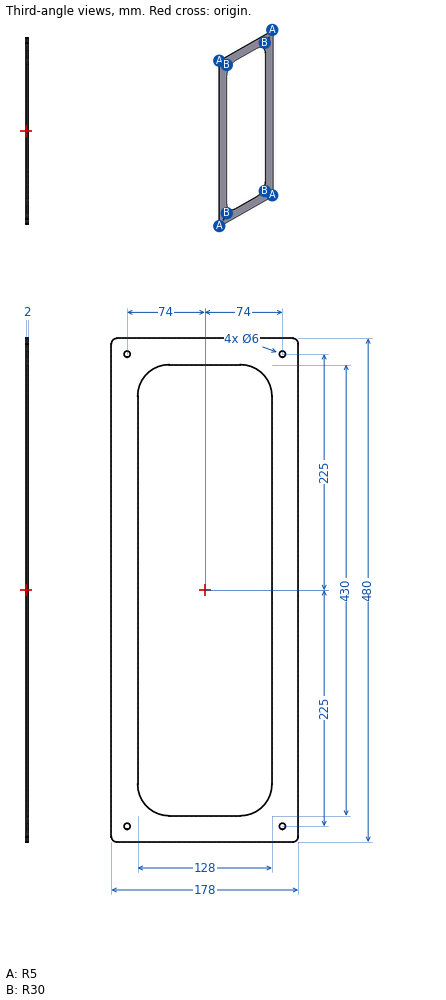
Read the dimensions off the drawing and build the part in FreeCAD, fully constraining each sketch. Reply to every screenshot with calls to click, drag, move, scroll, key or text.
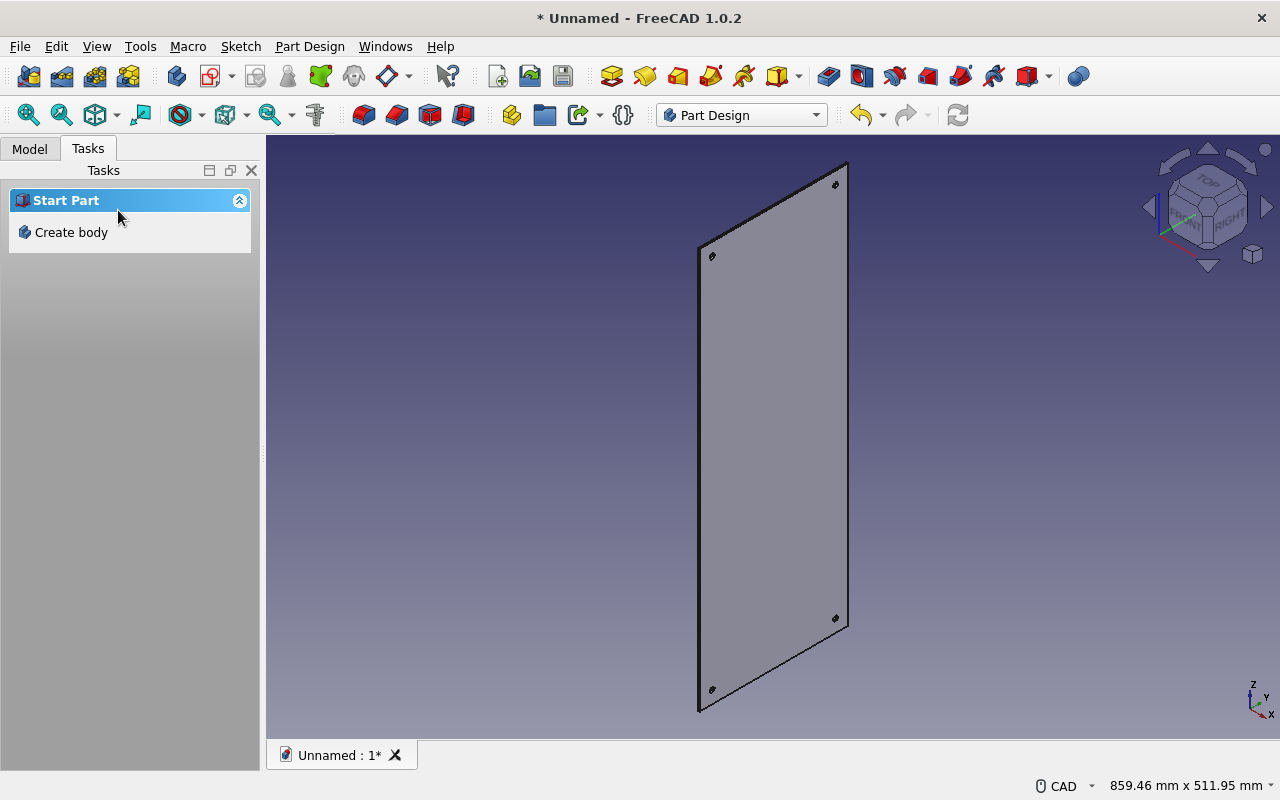
key(2)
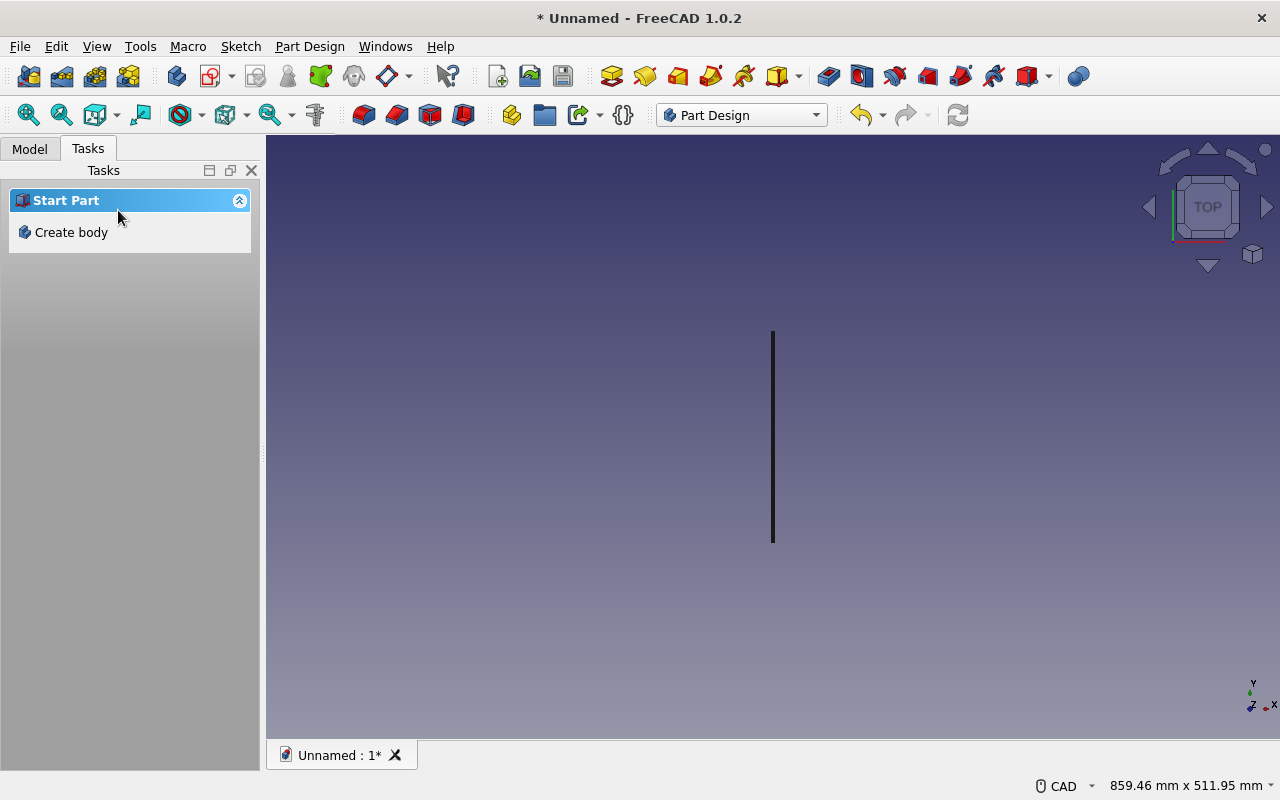
click(29, 116)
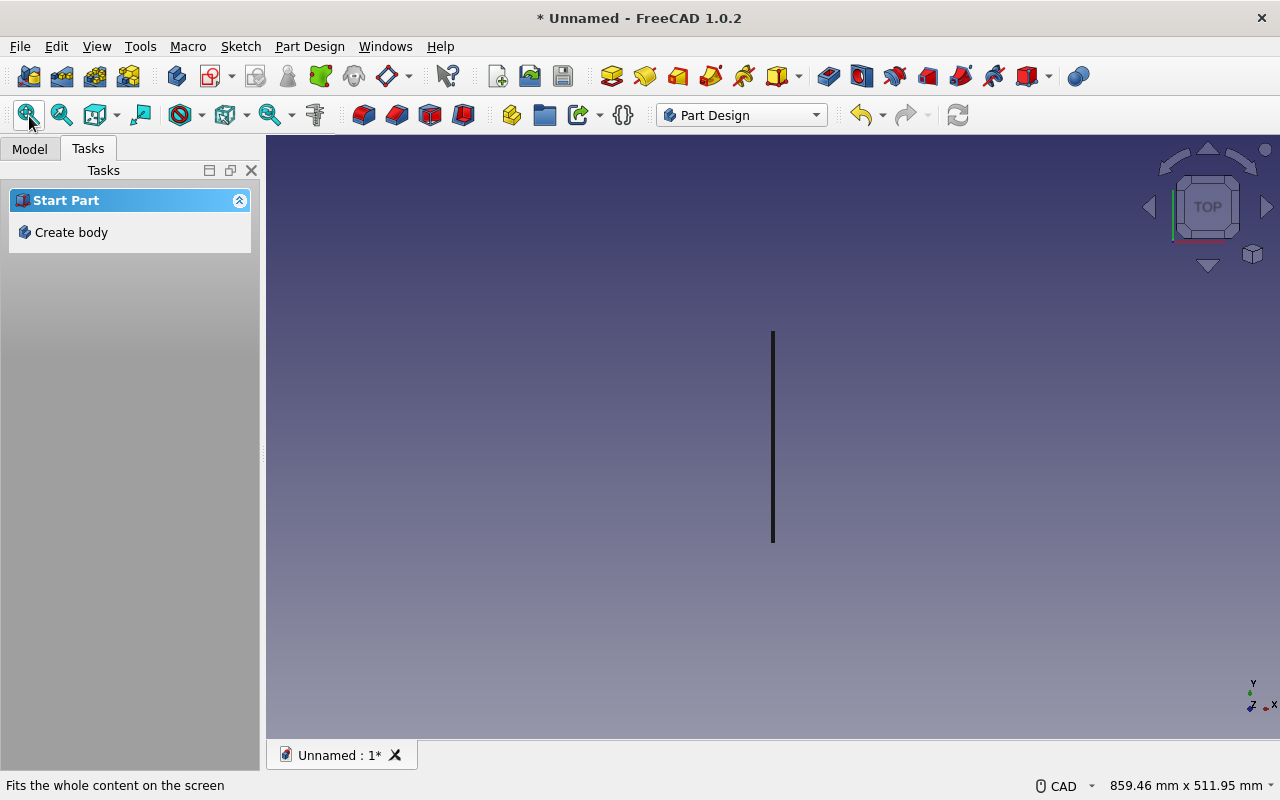
scroll(773, 331, up, 15)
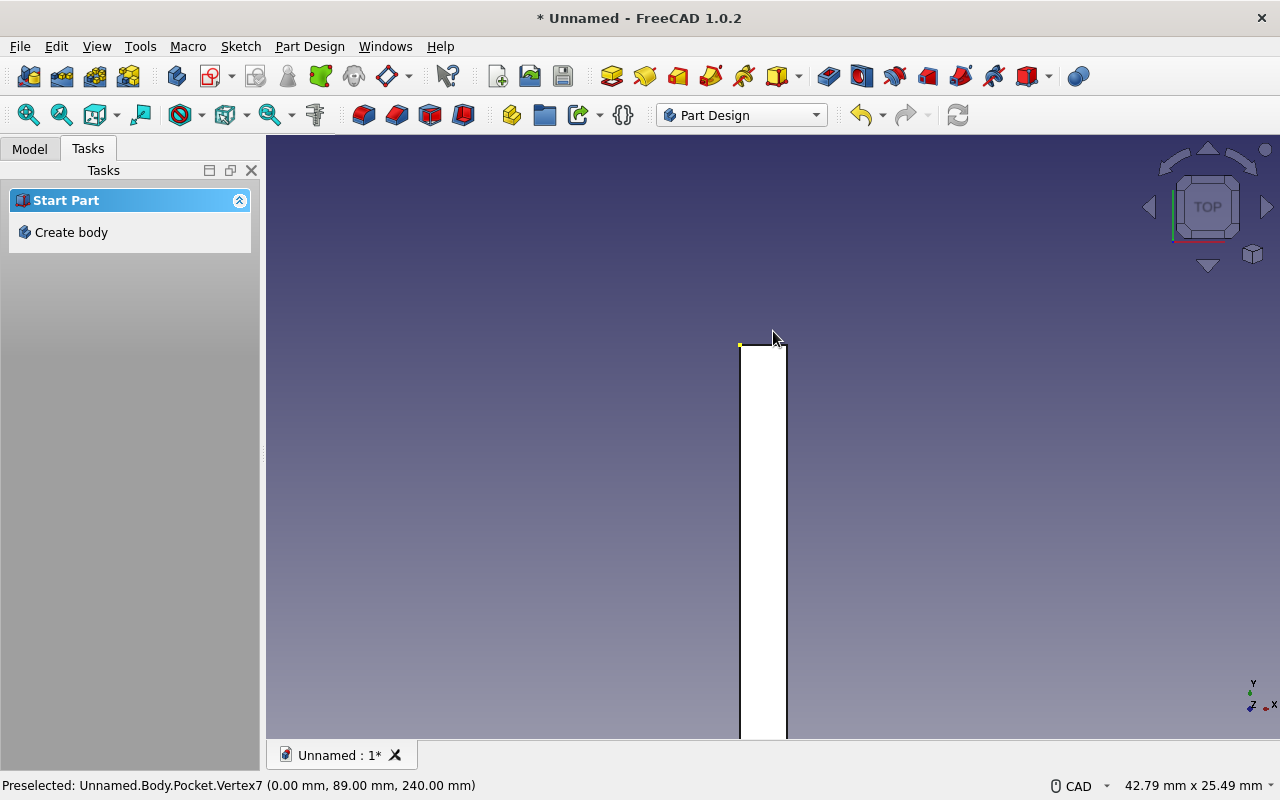
click(763, 344)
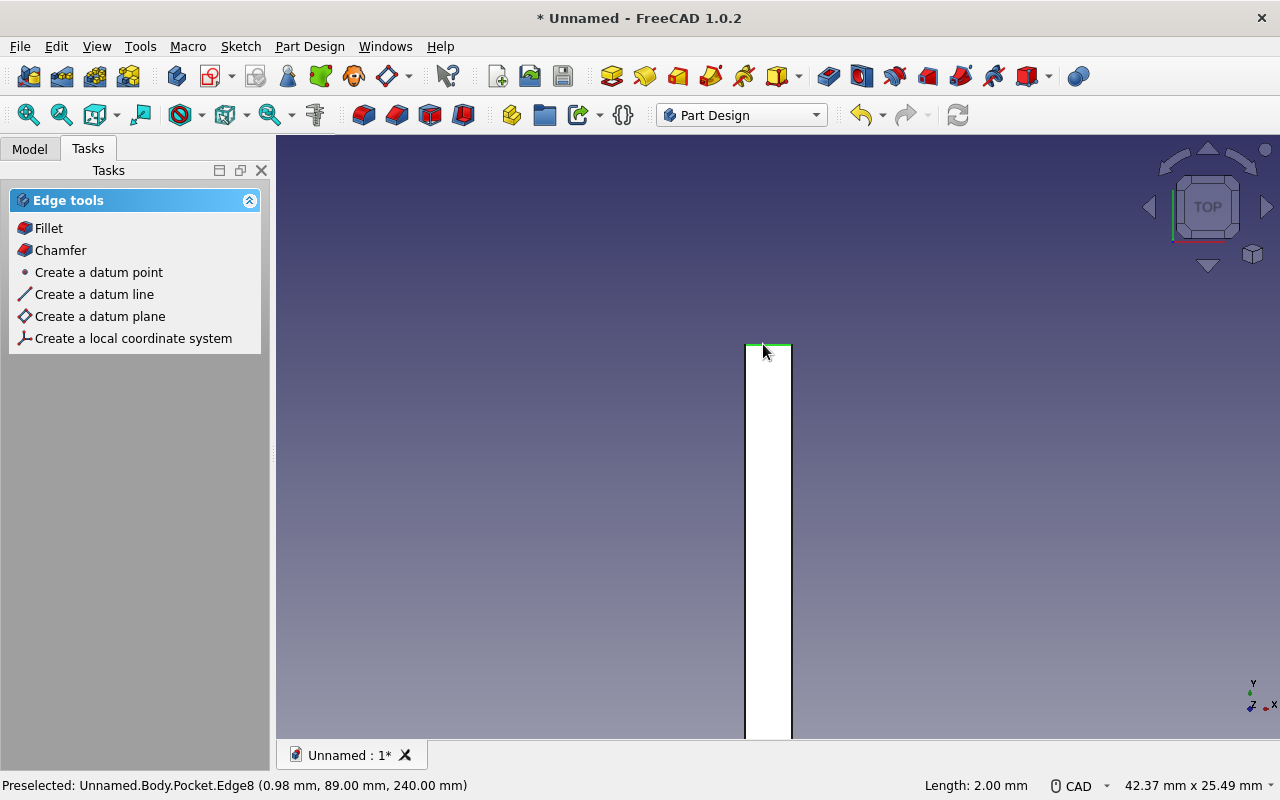
key(v)
key(f)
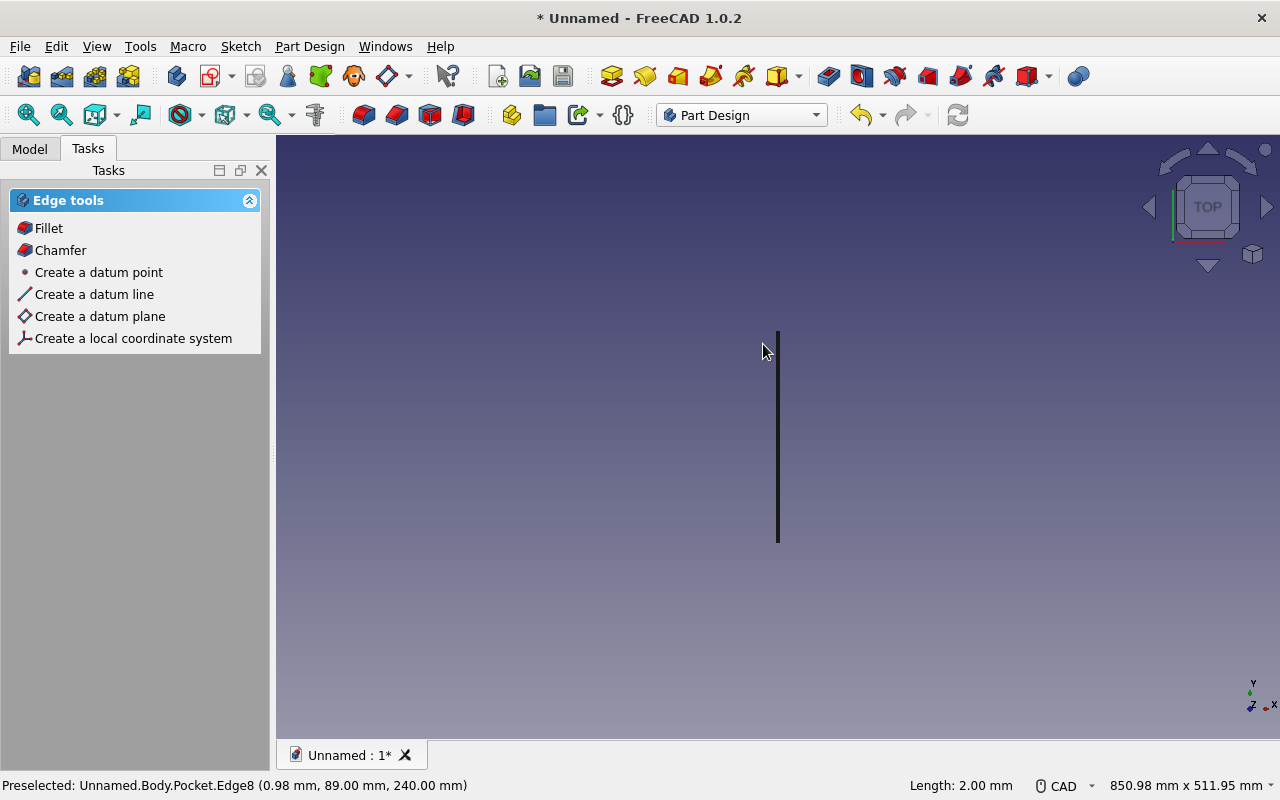
key(1)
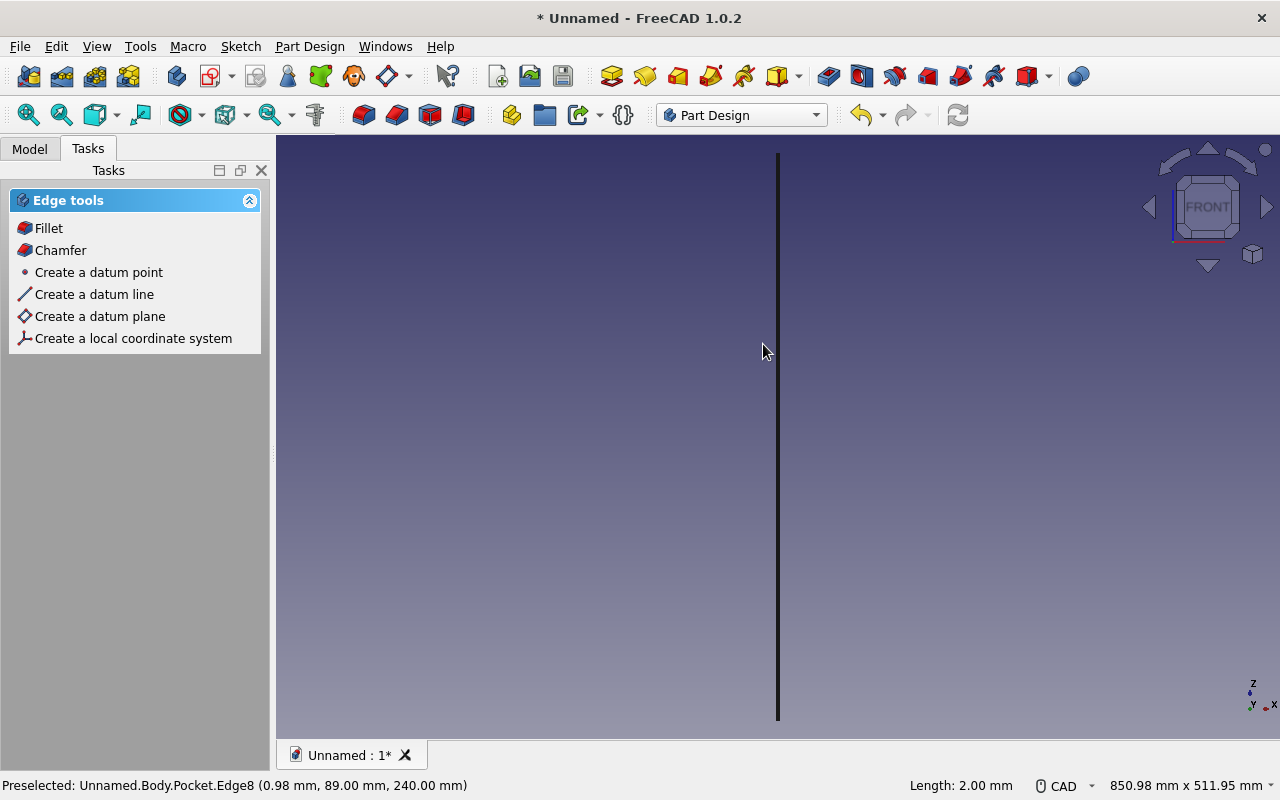
key(3)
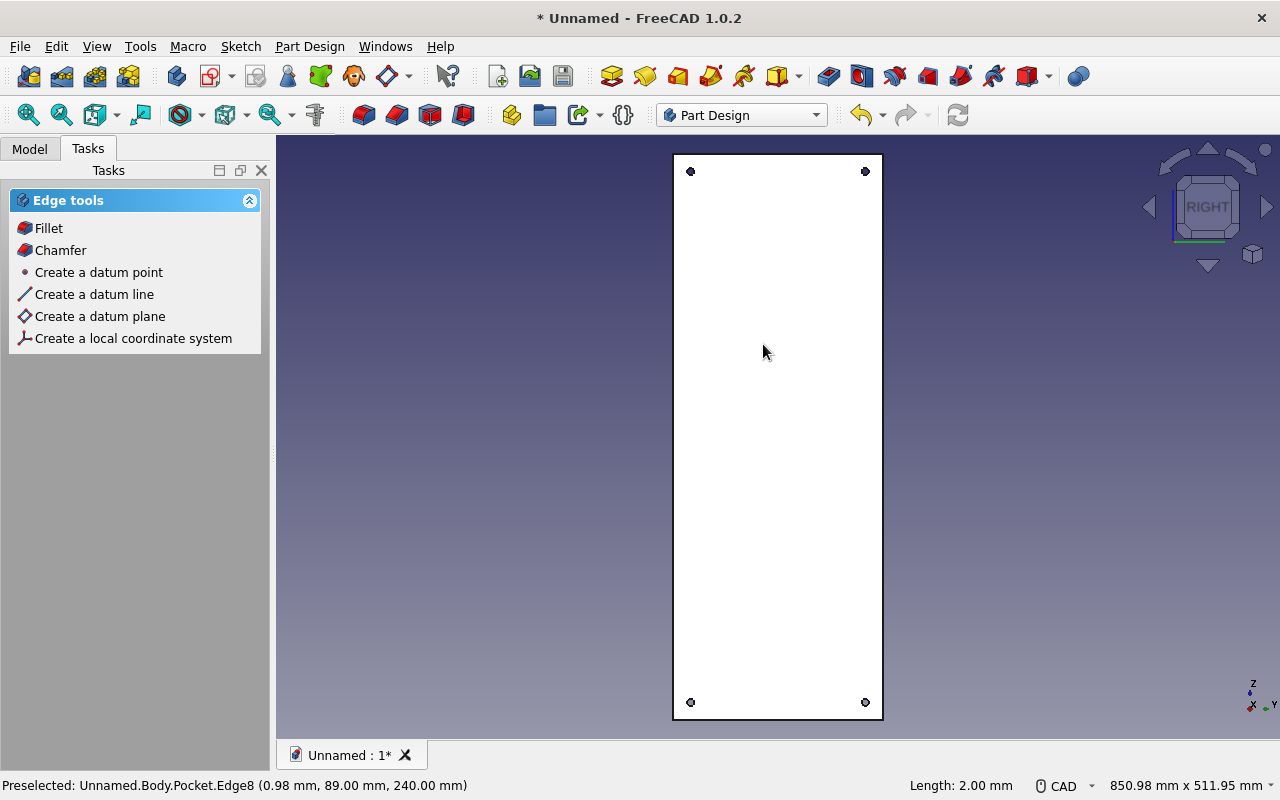
key(5)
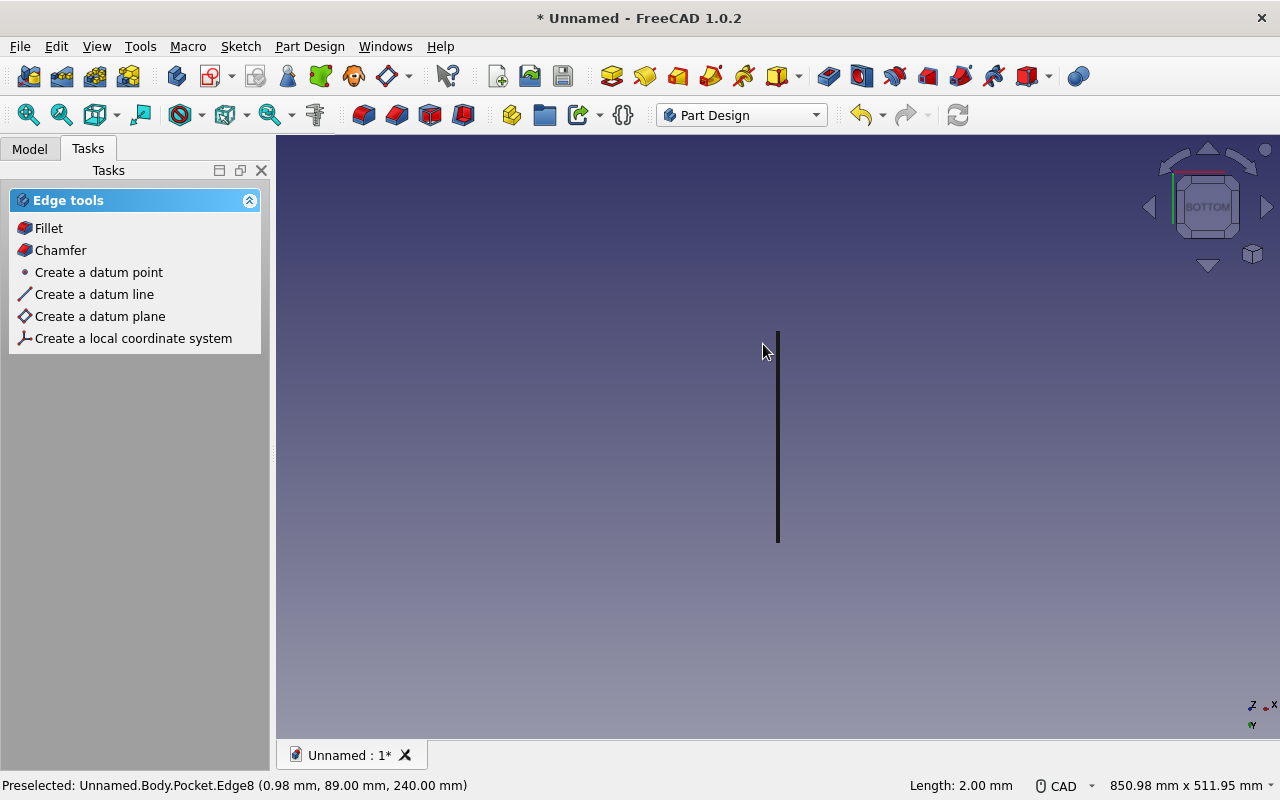
click(29, 116)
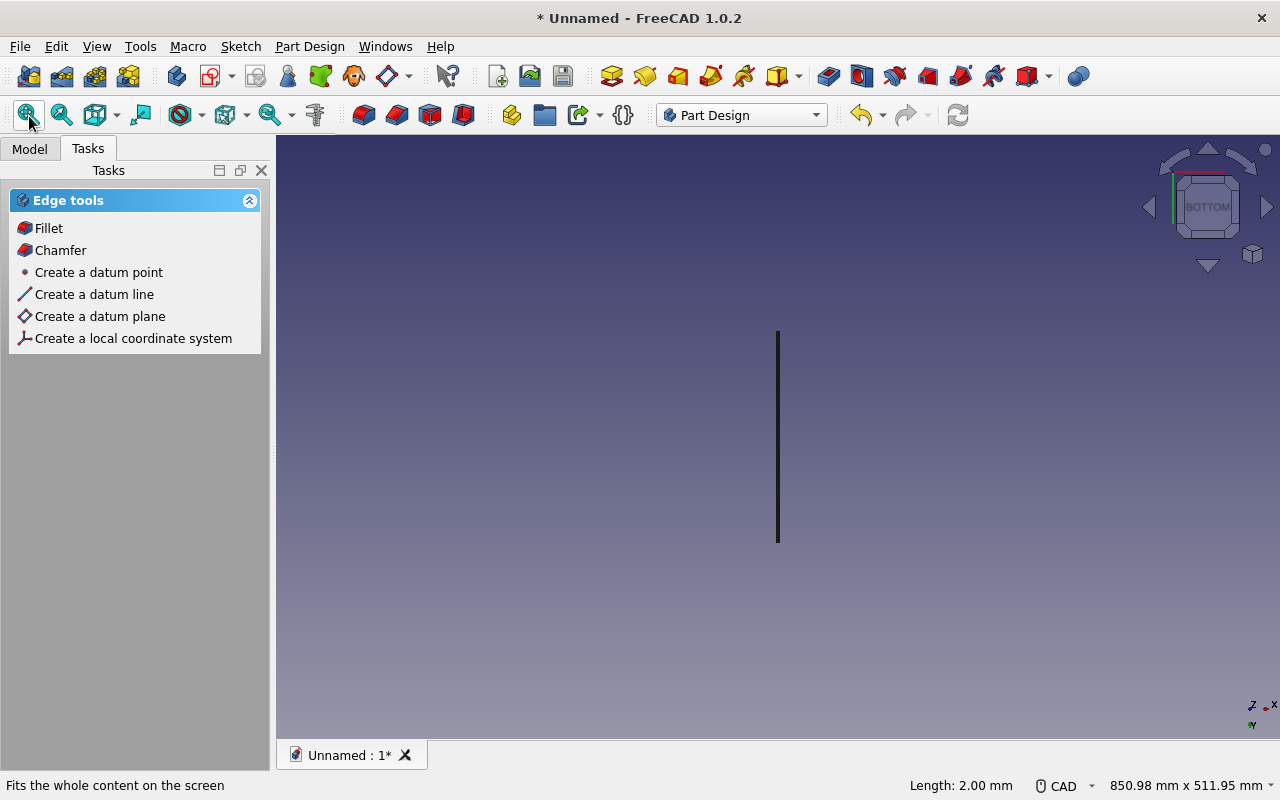
scroll(778, 541, up, 15)